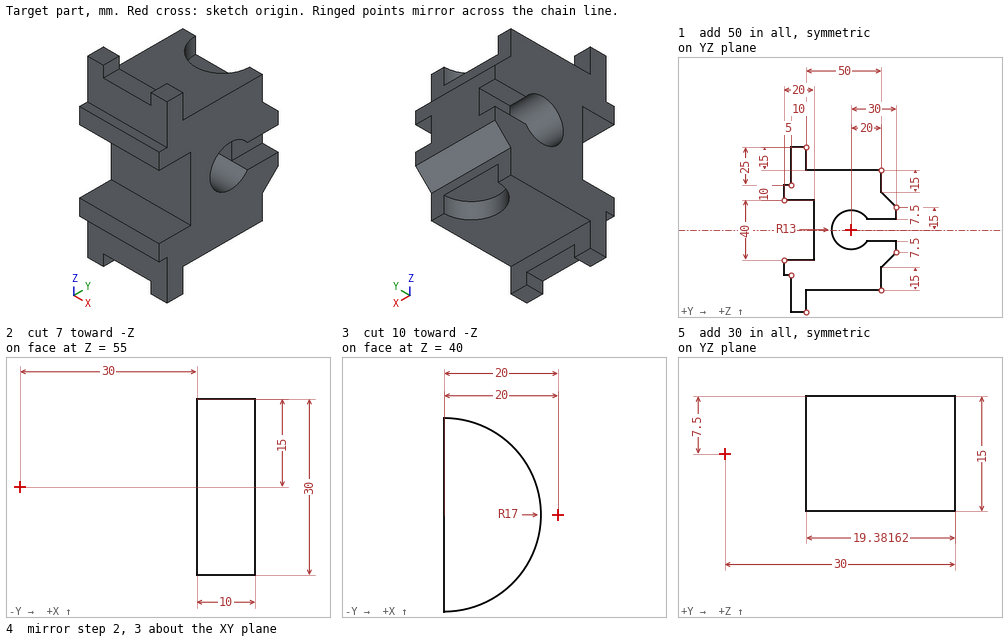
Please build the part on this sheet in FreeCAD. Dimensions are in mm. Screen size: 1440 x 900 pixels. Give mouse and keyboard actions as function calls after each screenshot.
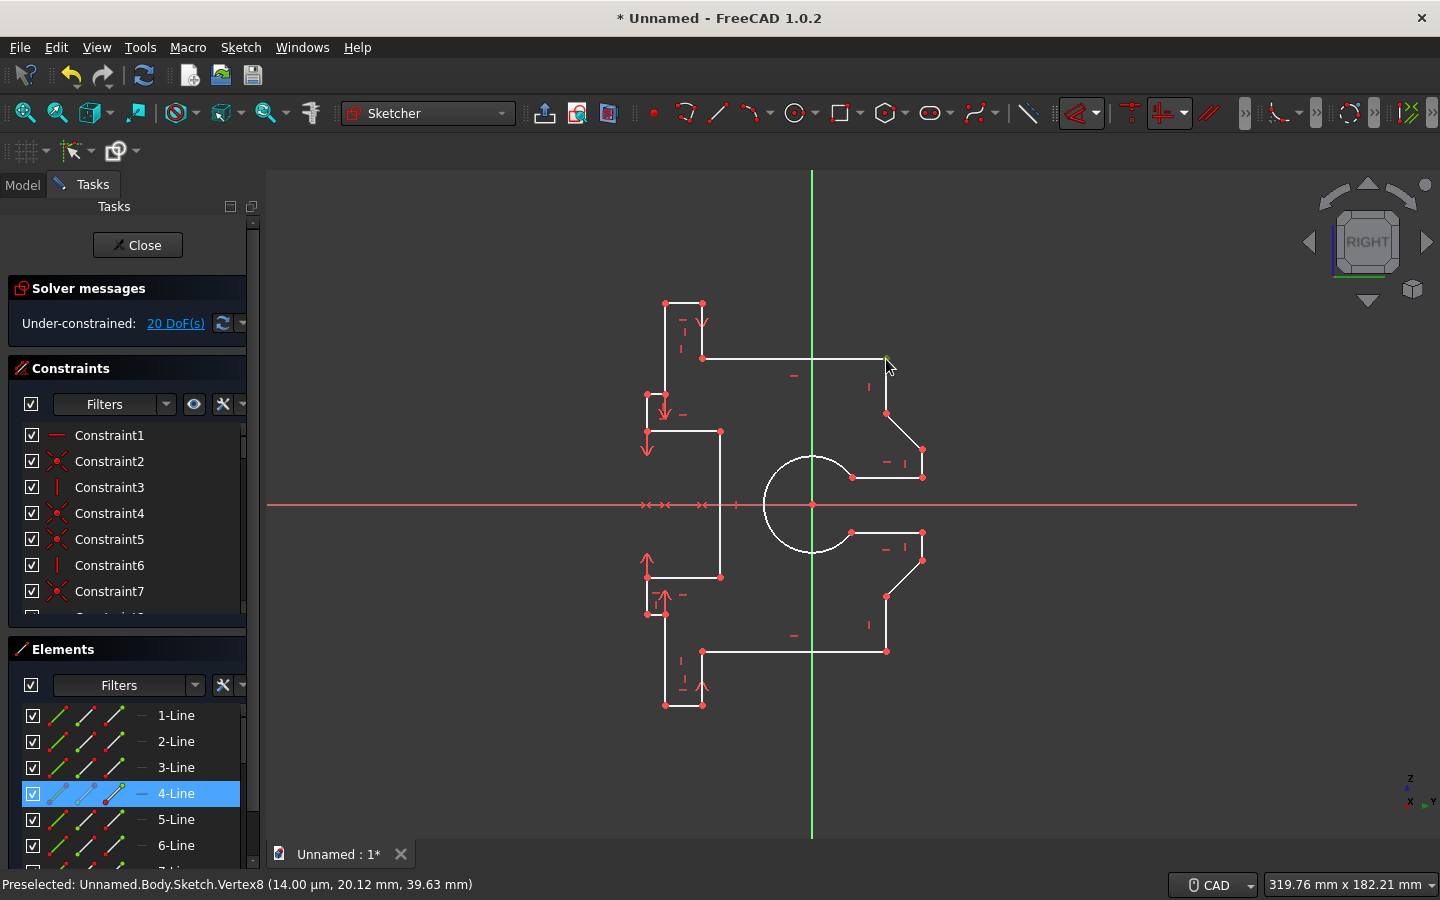
click(886, 652)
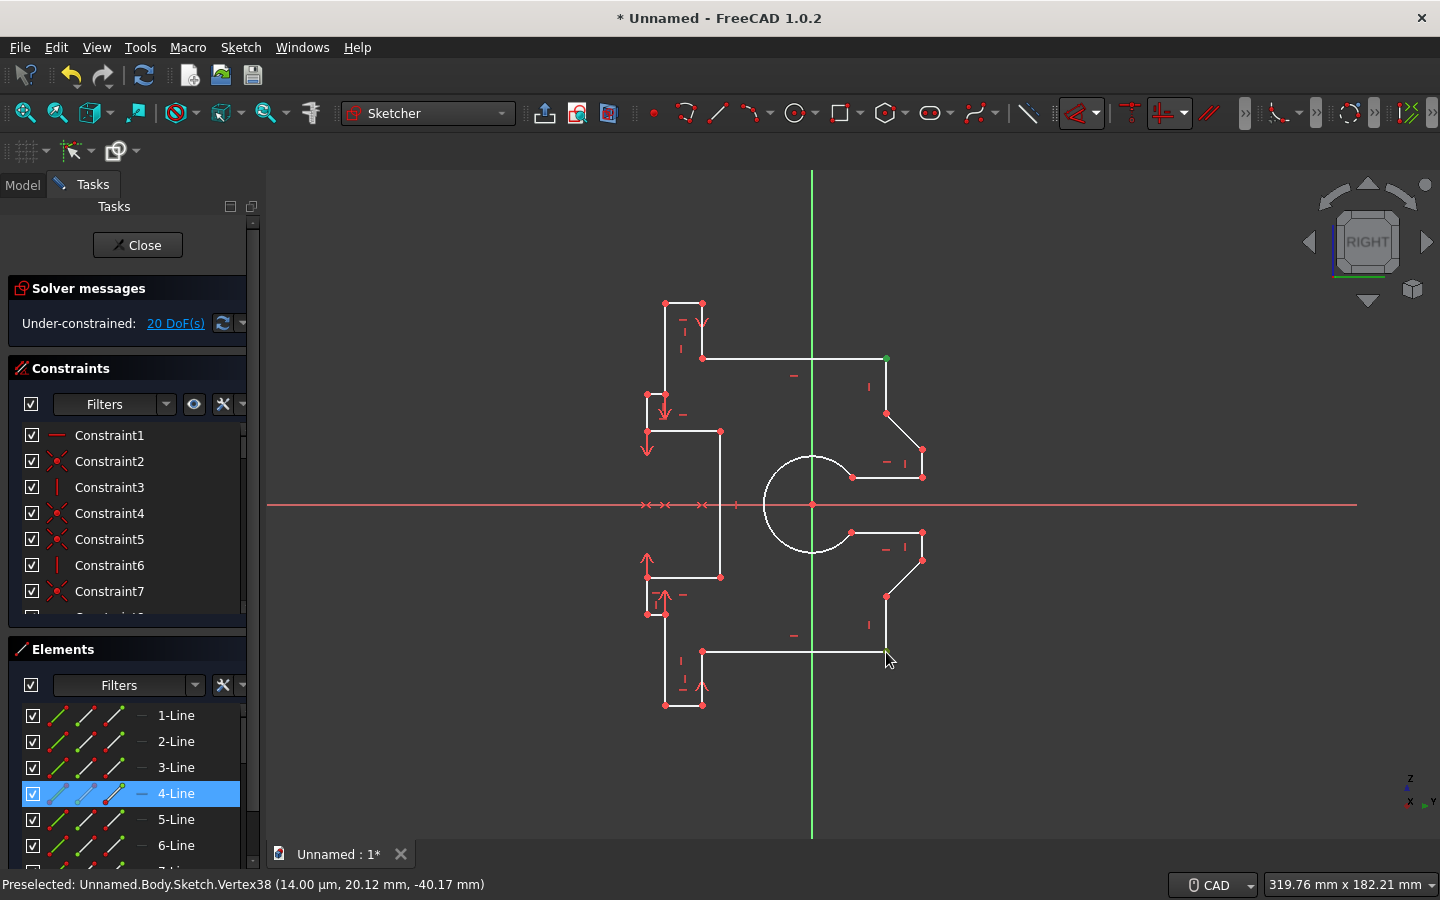
click(364, 504)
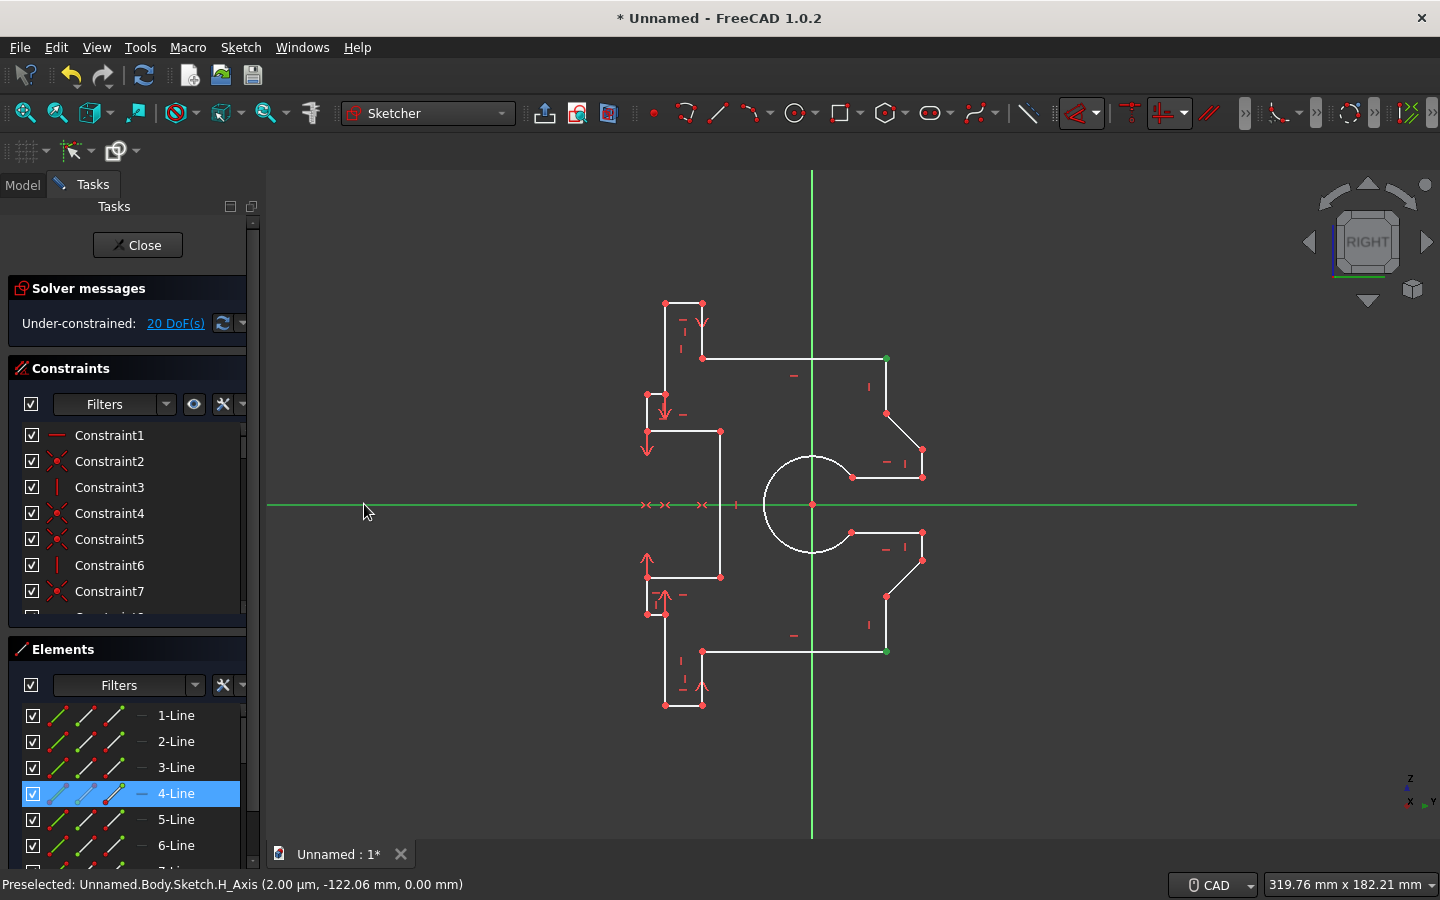
key(s)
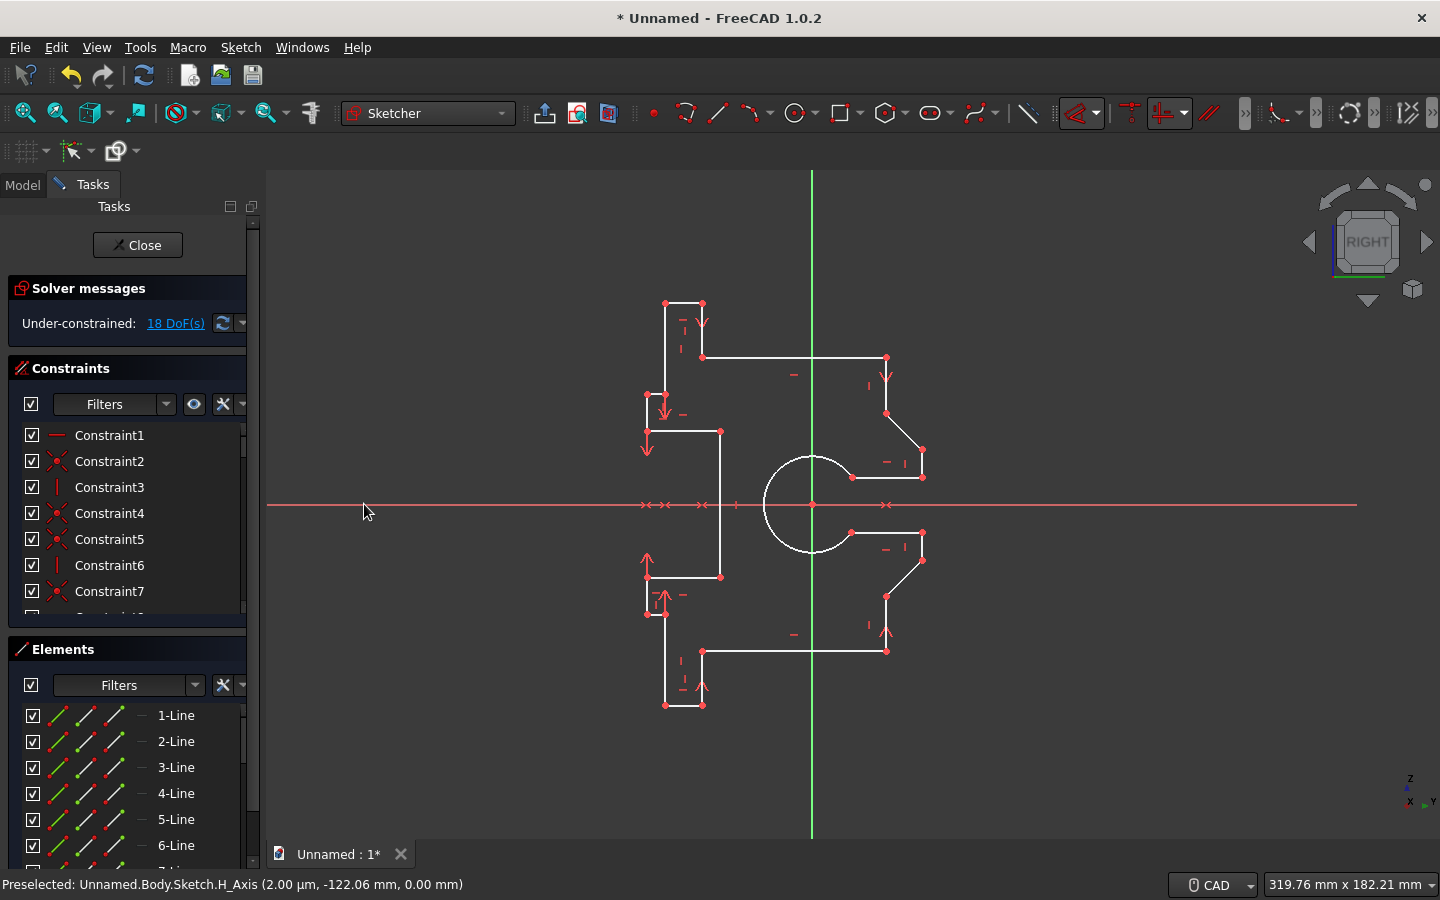
click(922, 450)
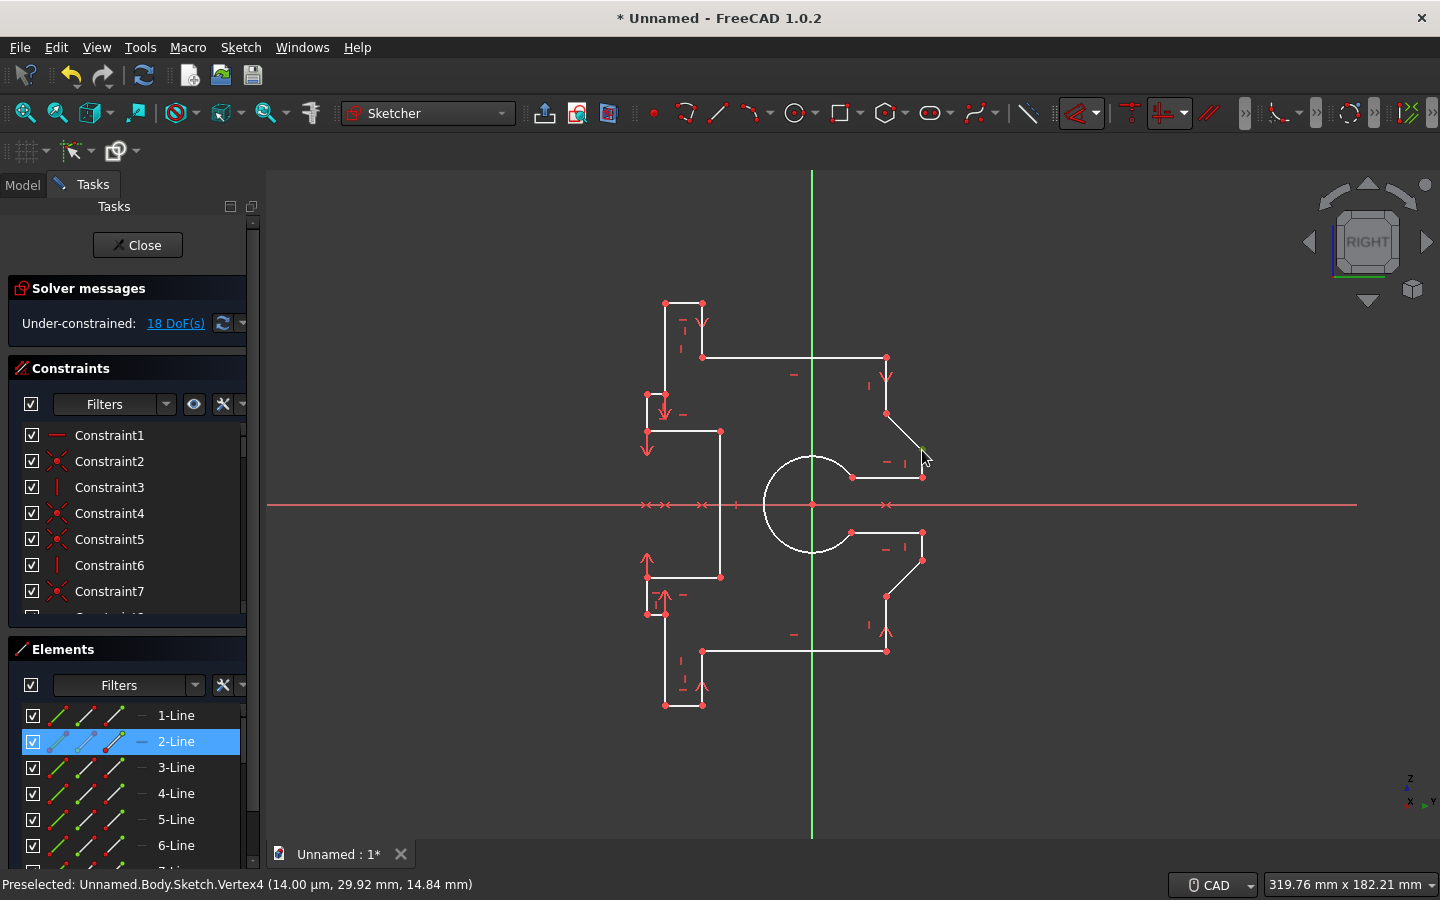
click(922, 561)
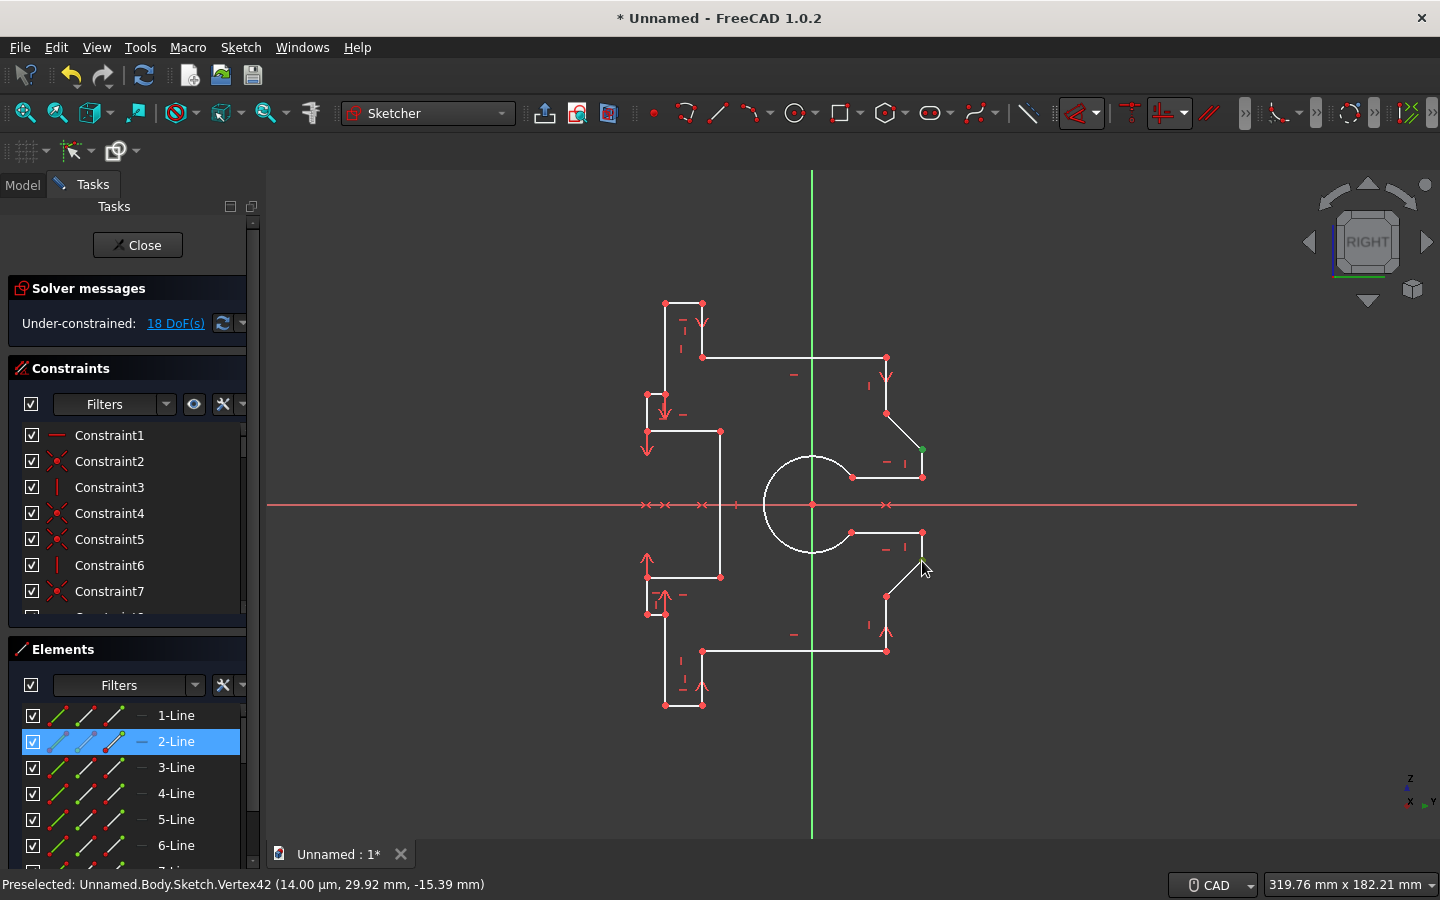
click(364, 504)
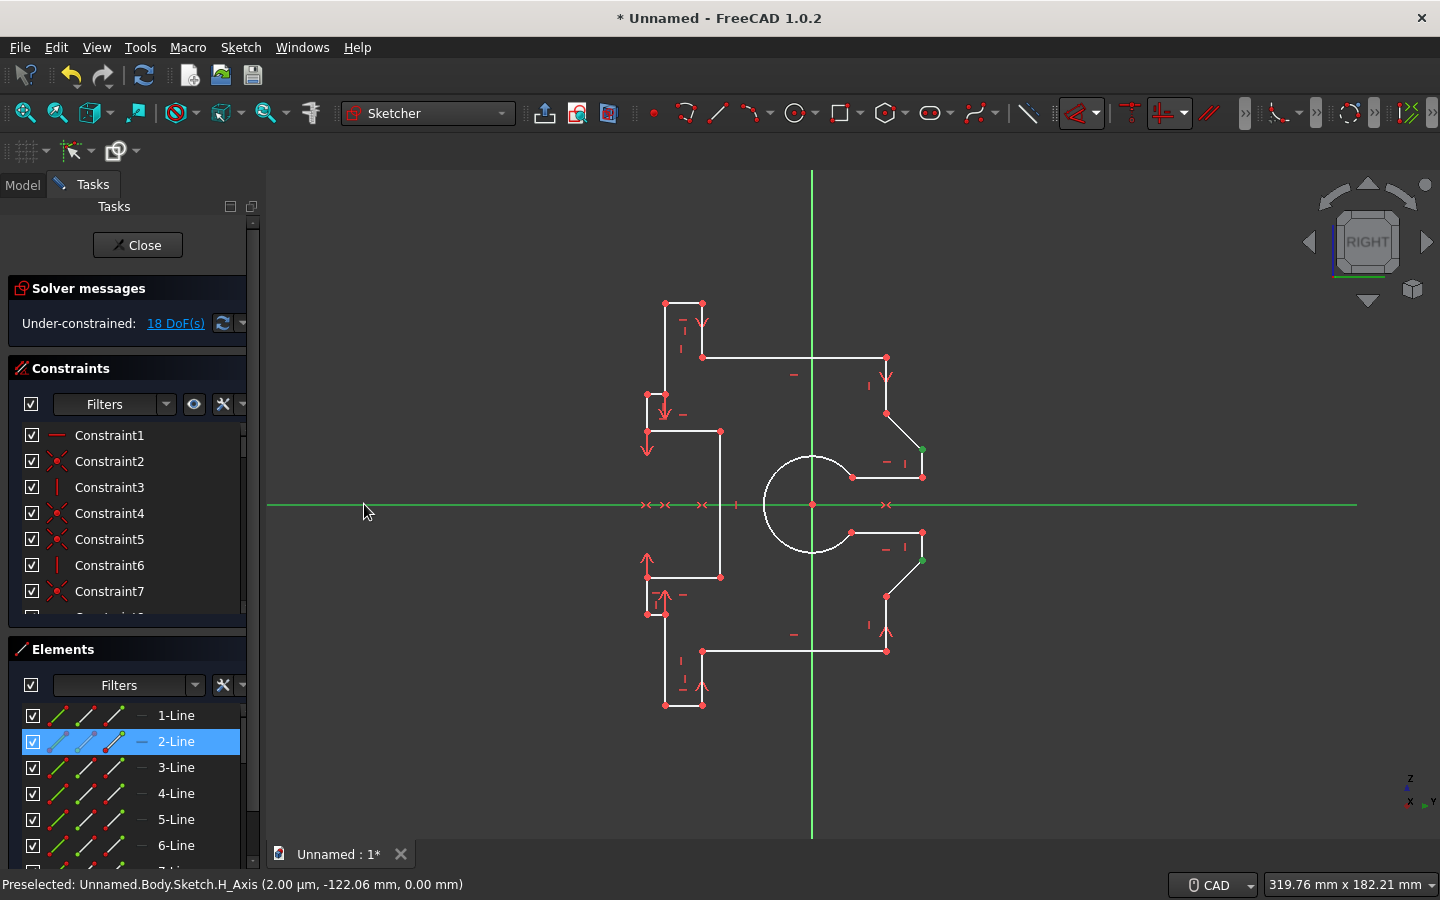
key(s)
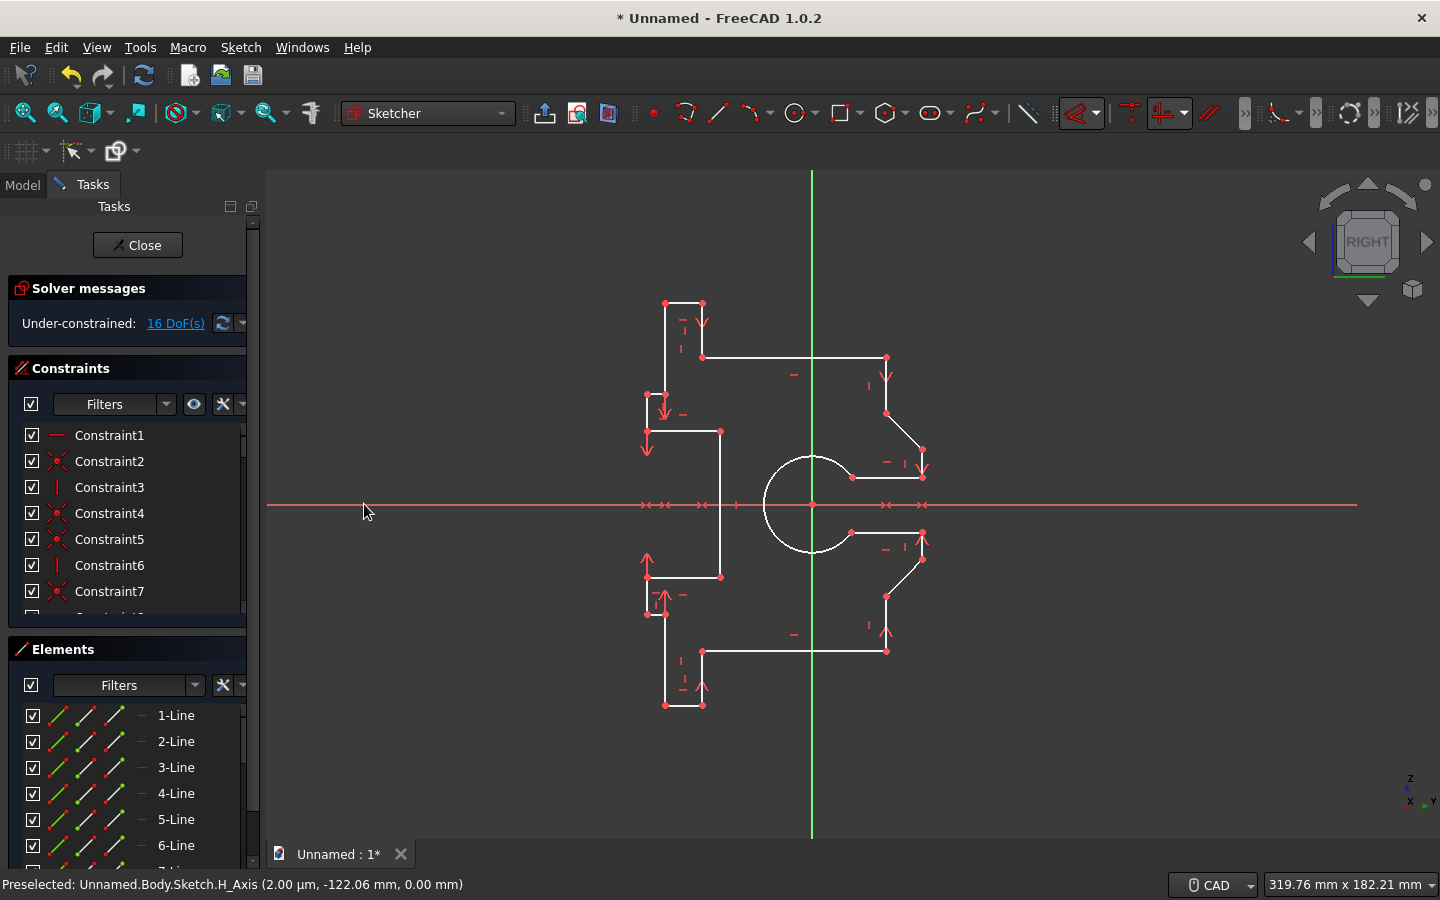
click(1076, 114)